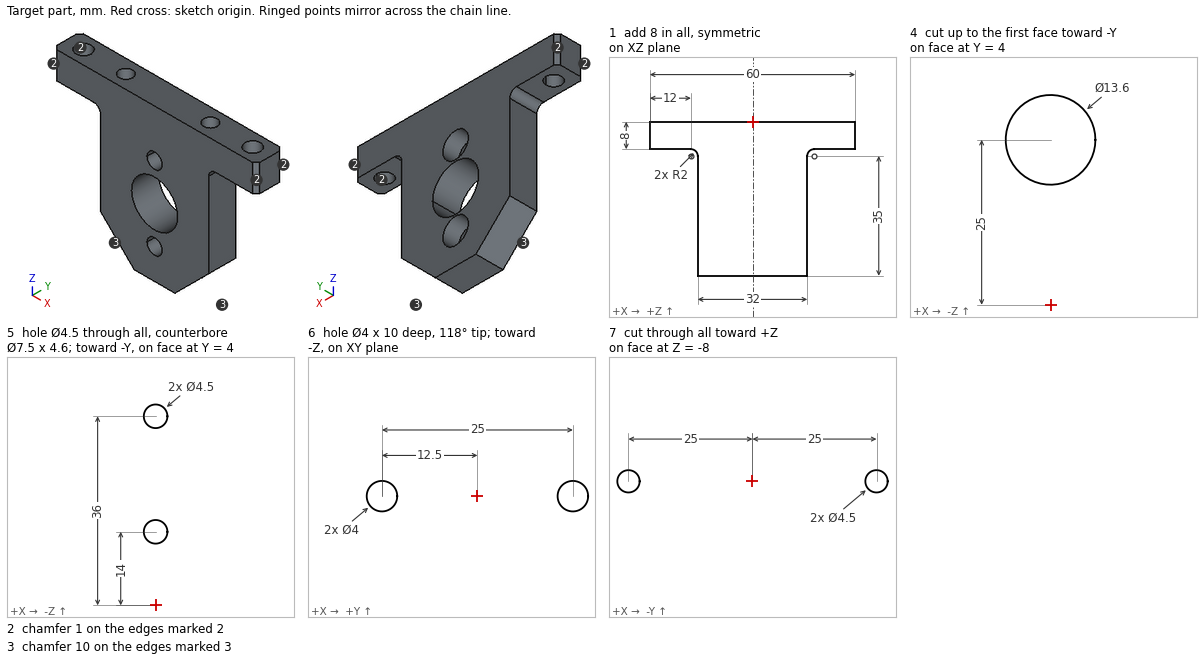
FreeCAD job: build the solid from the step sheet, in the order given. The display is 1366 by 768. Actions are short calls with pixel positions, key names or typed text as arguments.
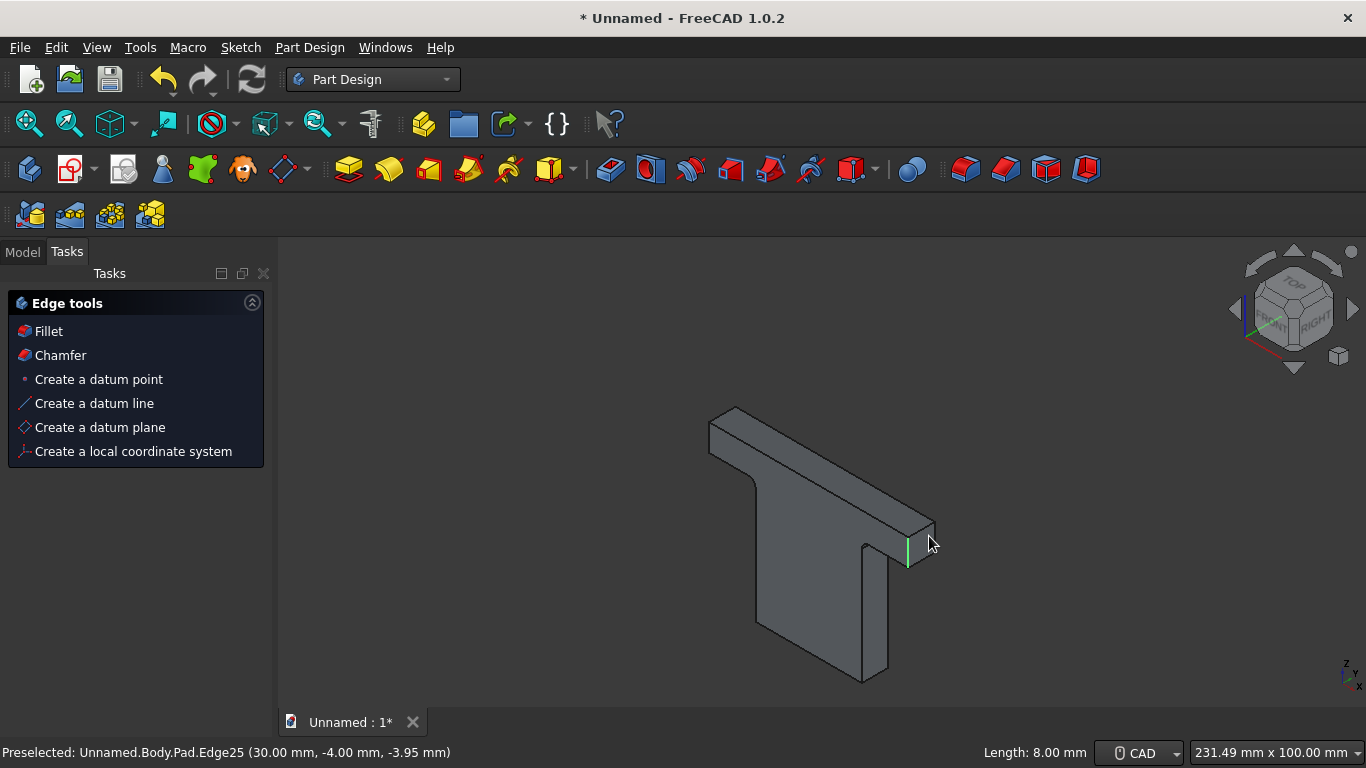
key(v)
key(f)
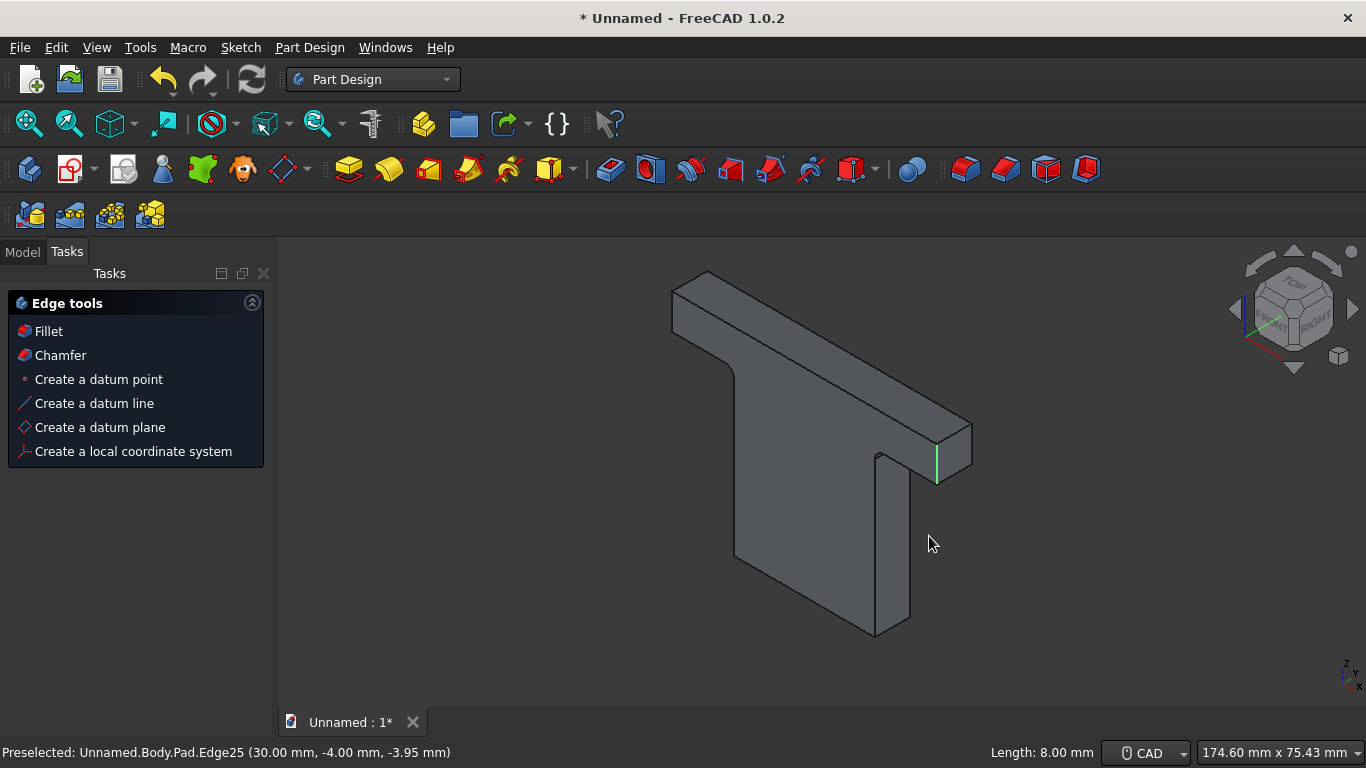
key(2)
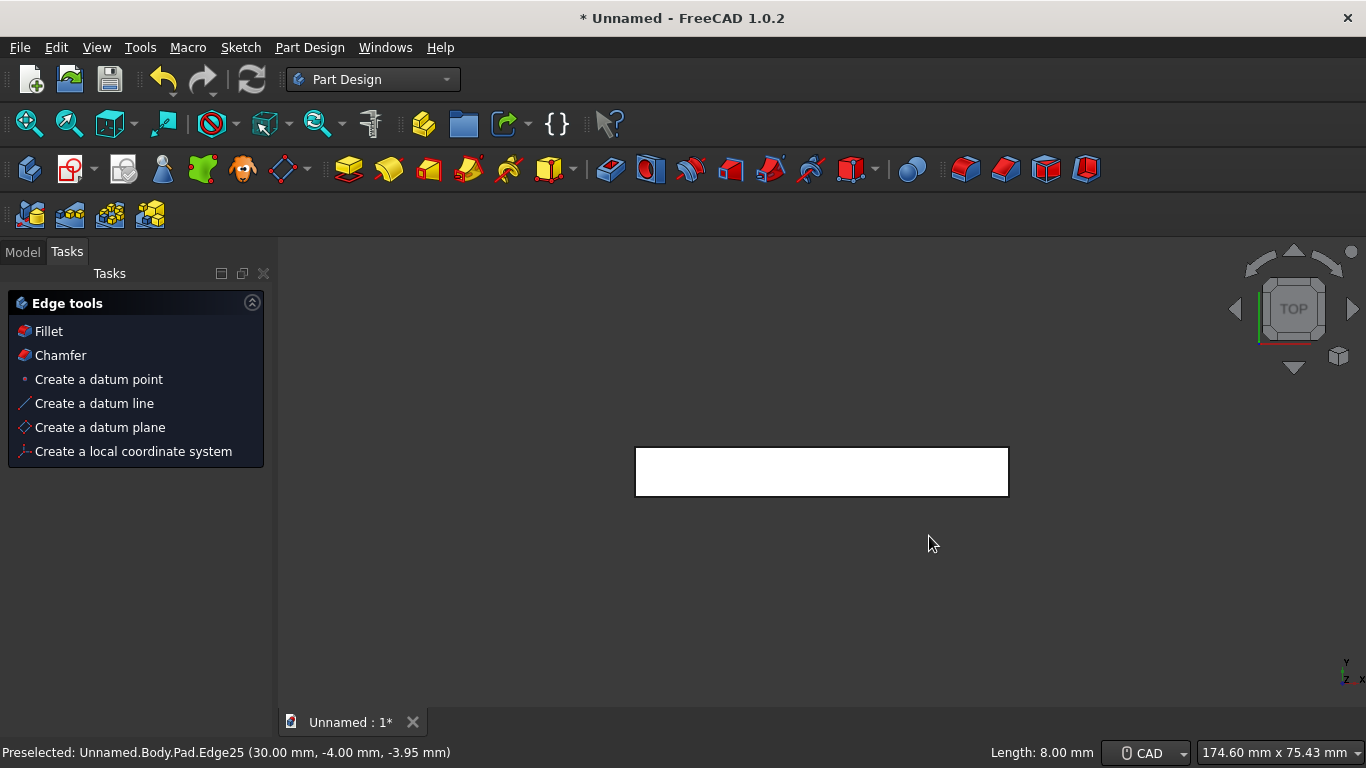
click(30, 124)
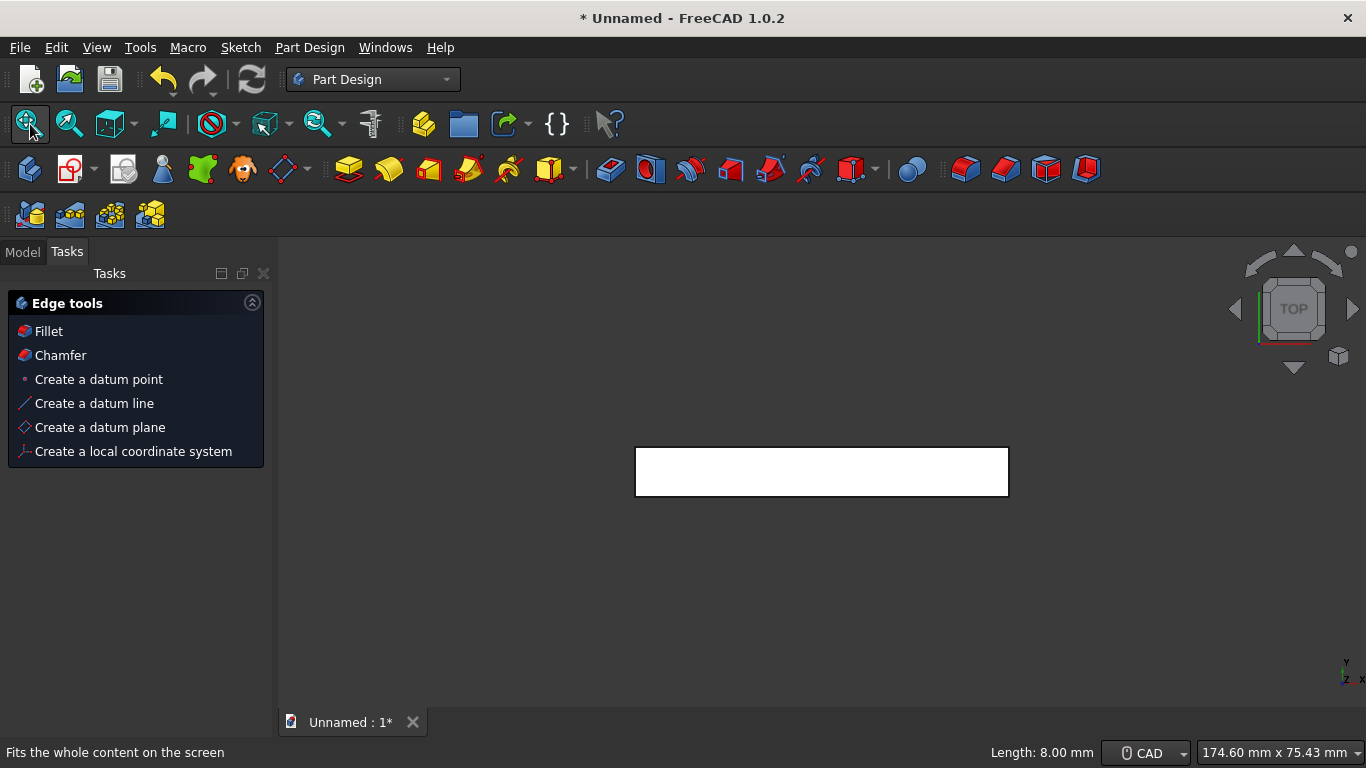
key(1)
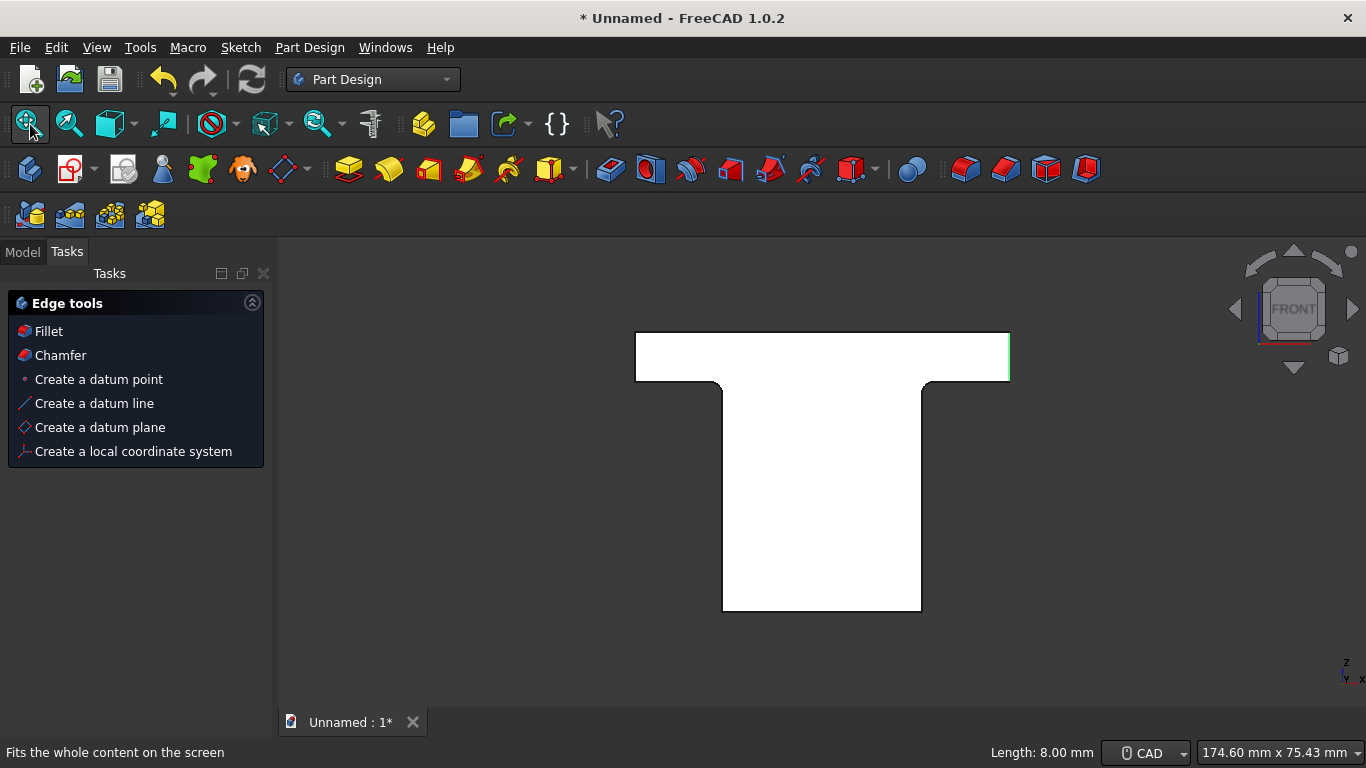
click(635, 356, ctrl)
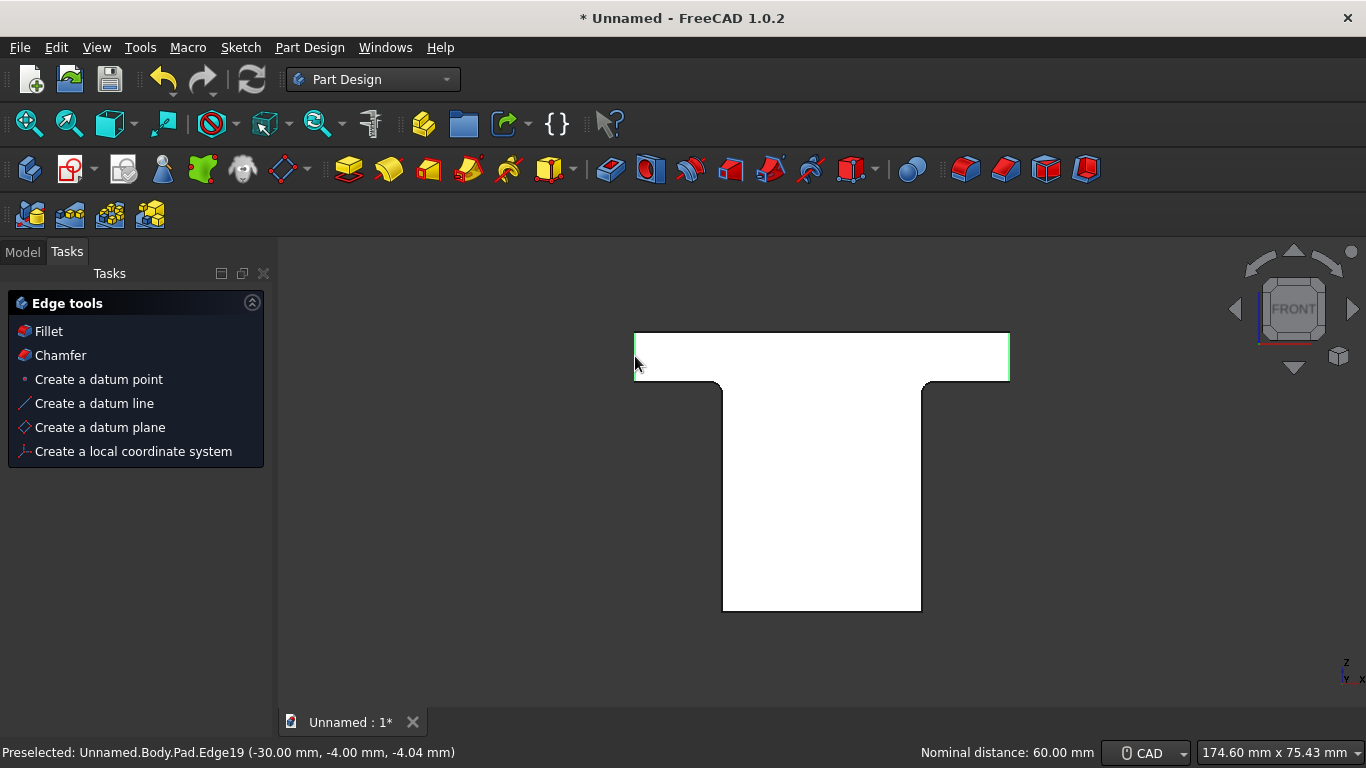
key(3)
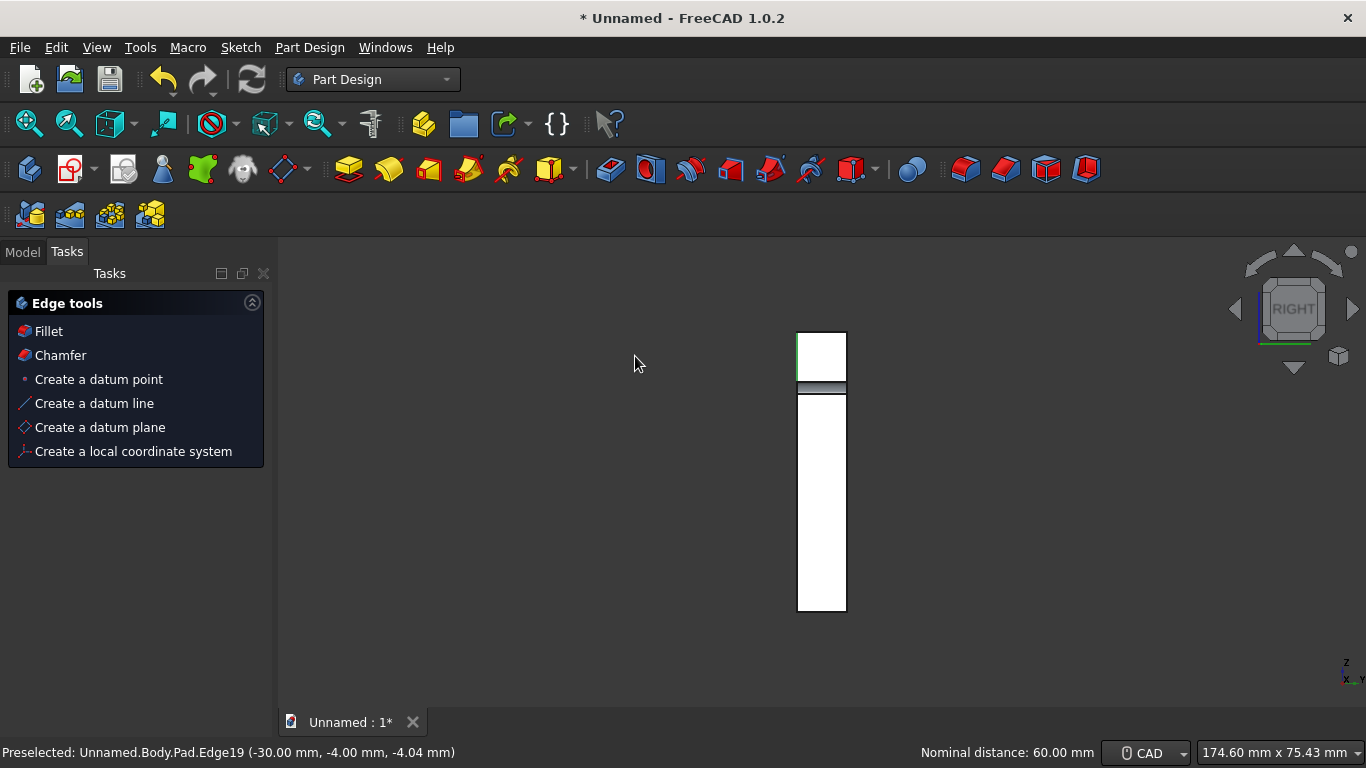
click(847, 356, ctrl)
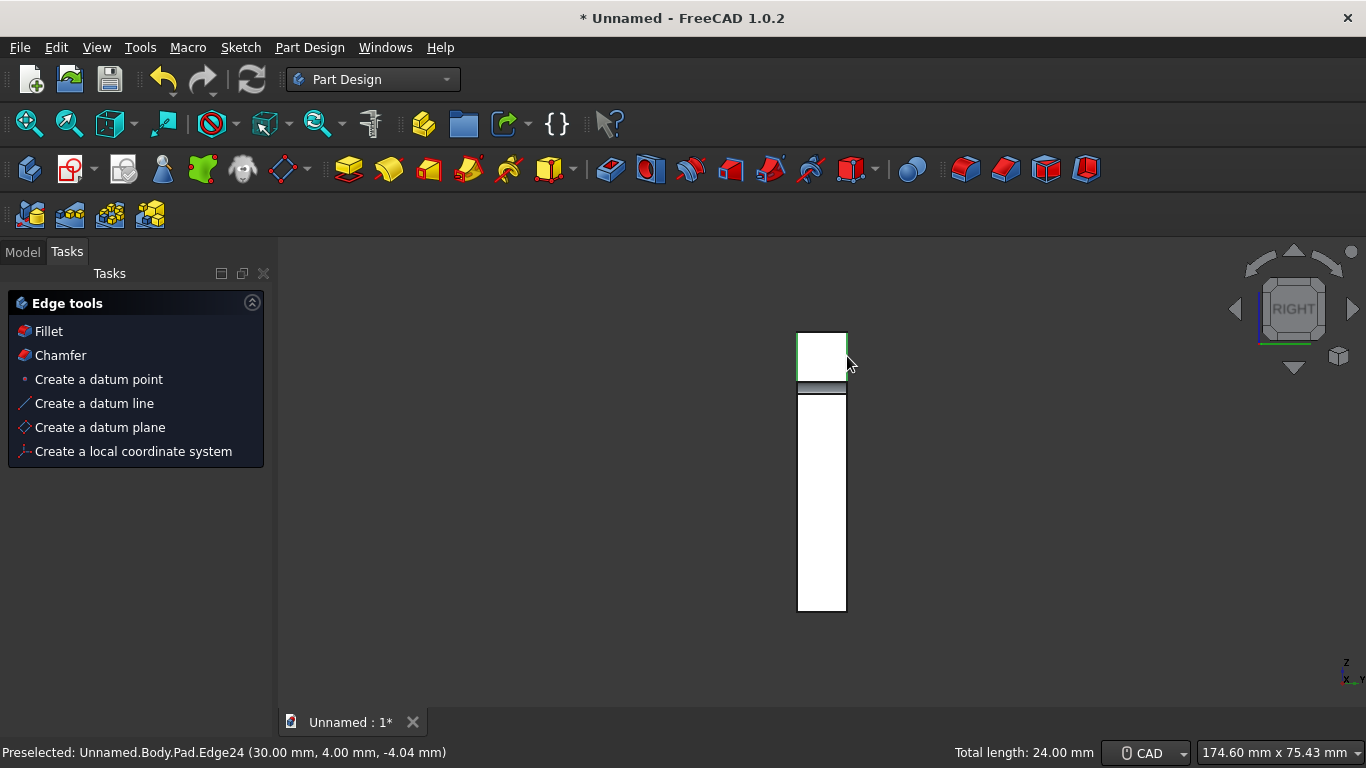
key(5)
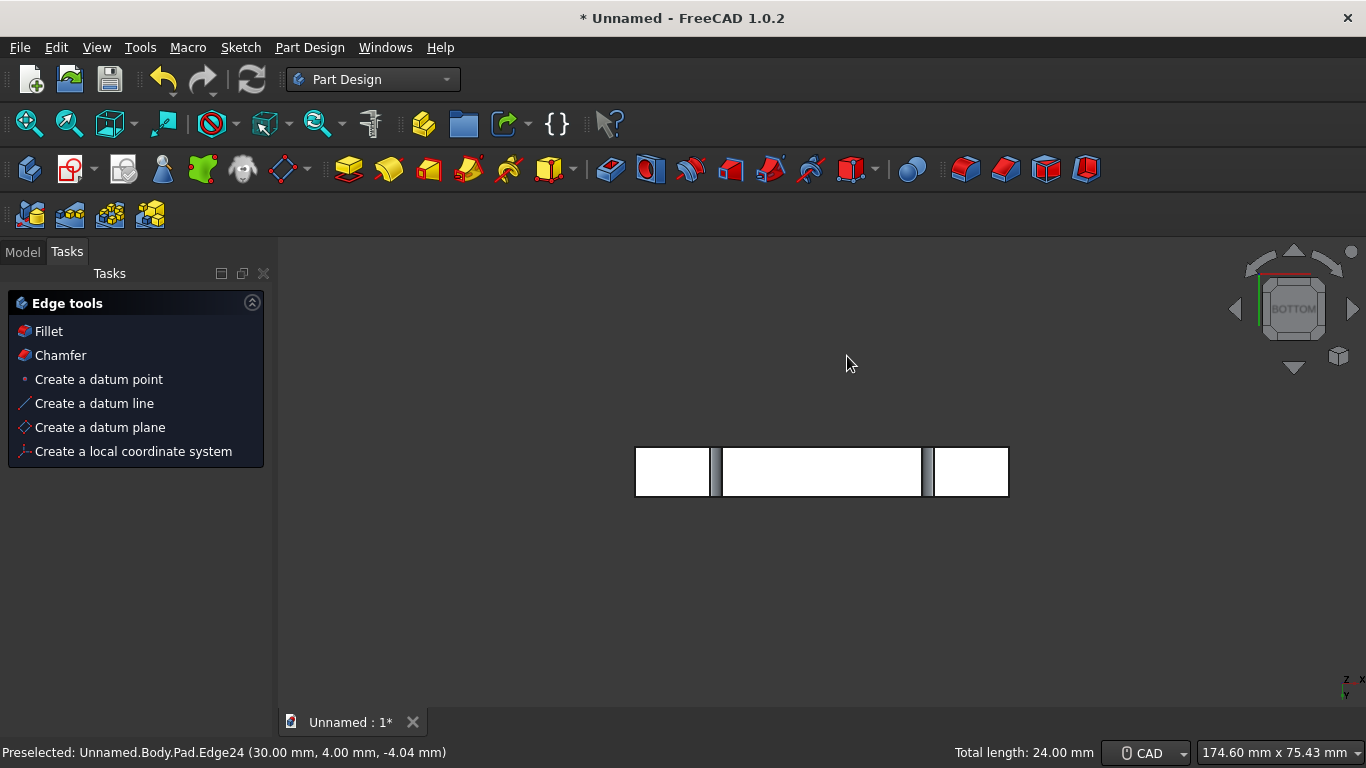
click(30, 124)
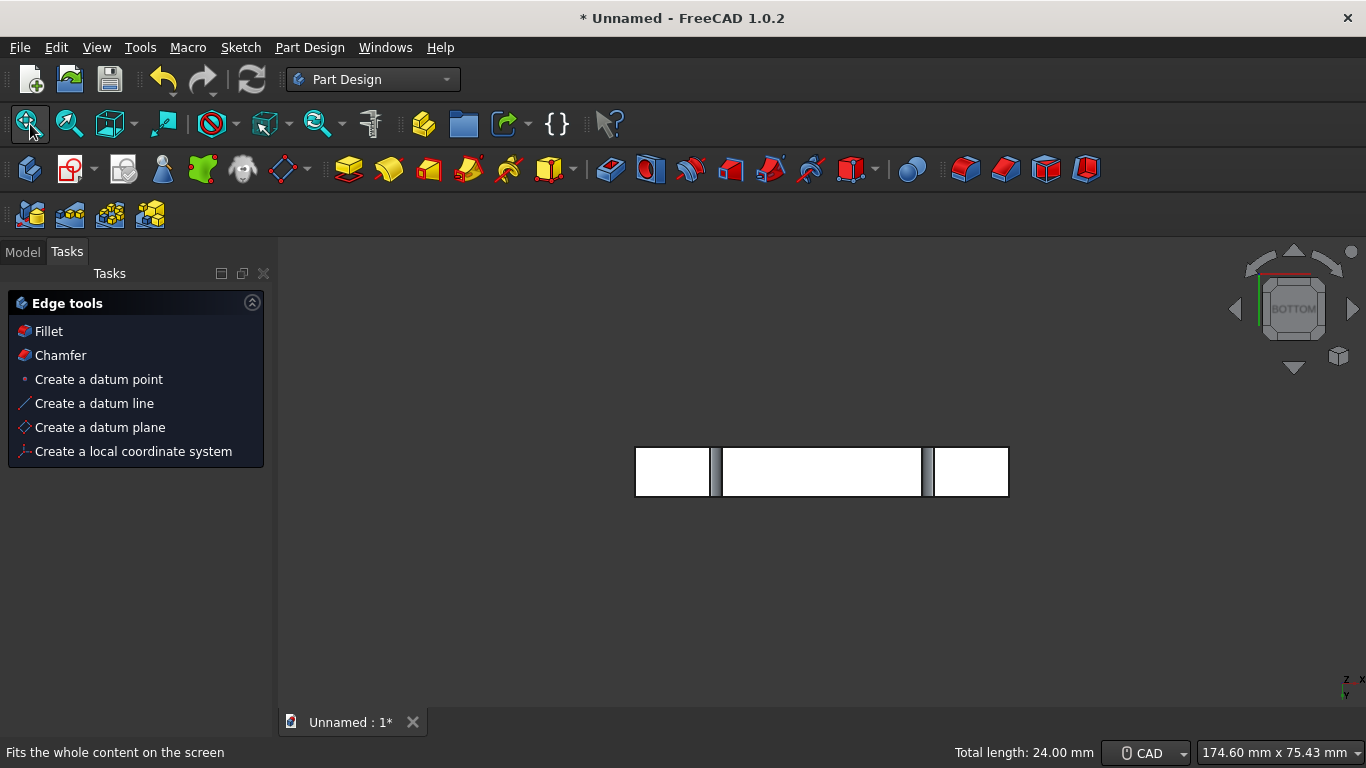
key(4)